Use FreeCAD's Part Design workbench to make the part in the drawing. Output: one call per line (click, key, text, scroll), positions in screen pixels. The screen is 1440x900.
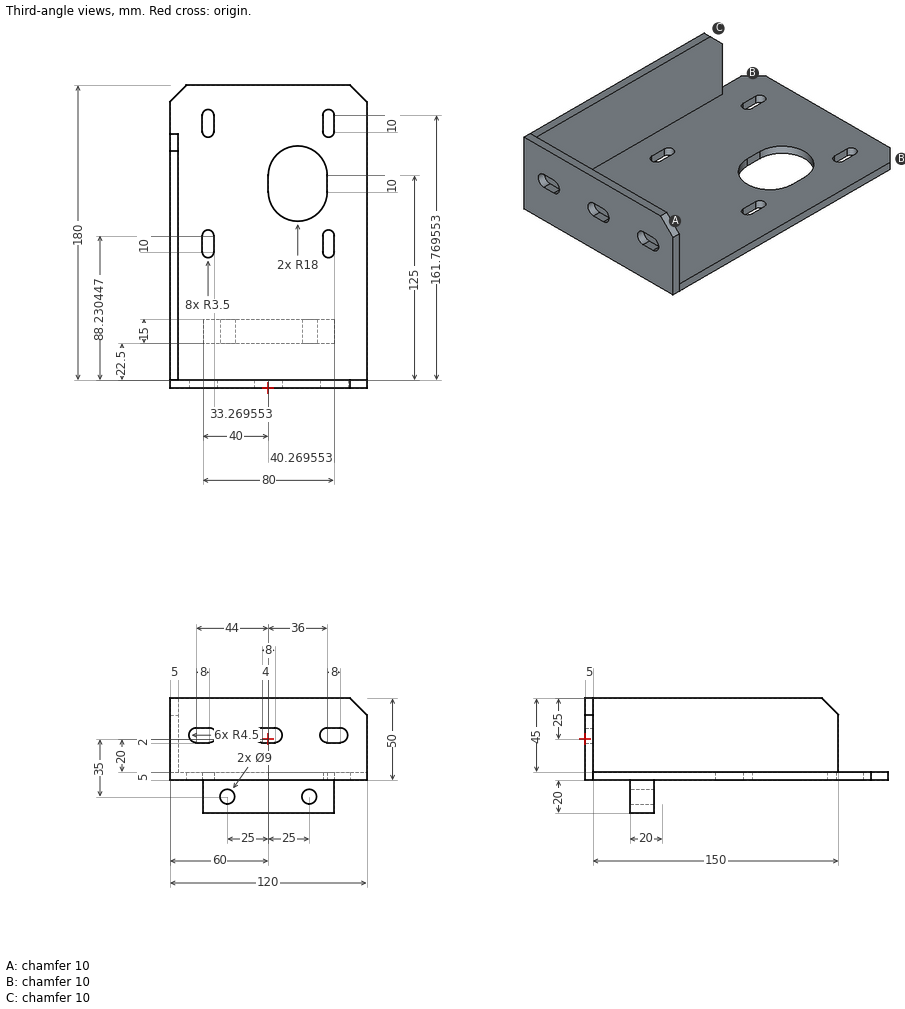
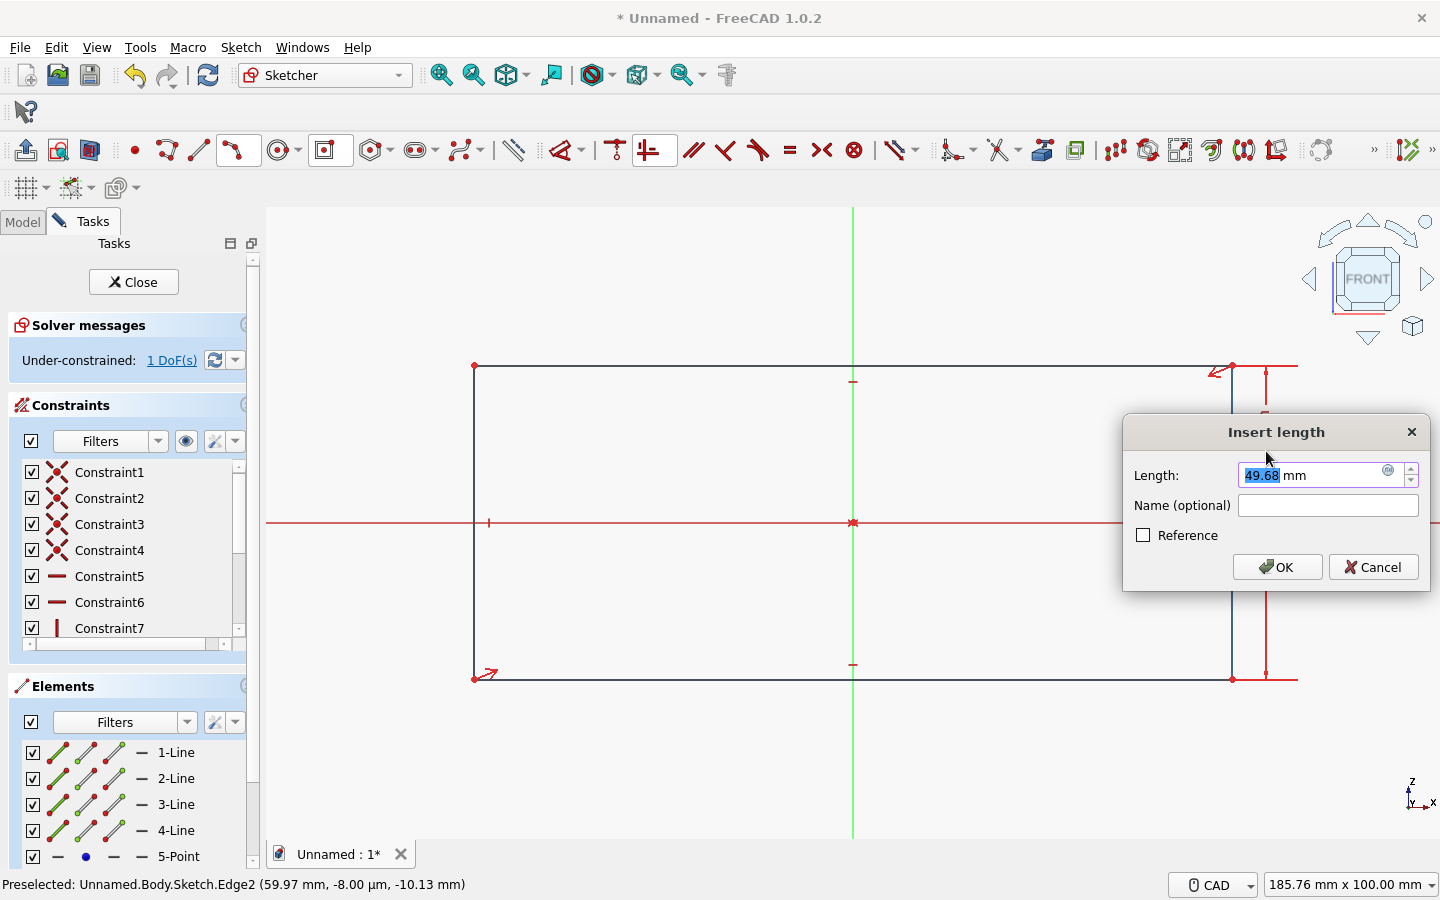
text(50)
key(Return)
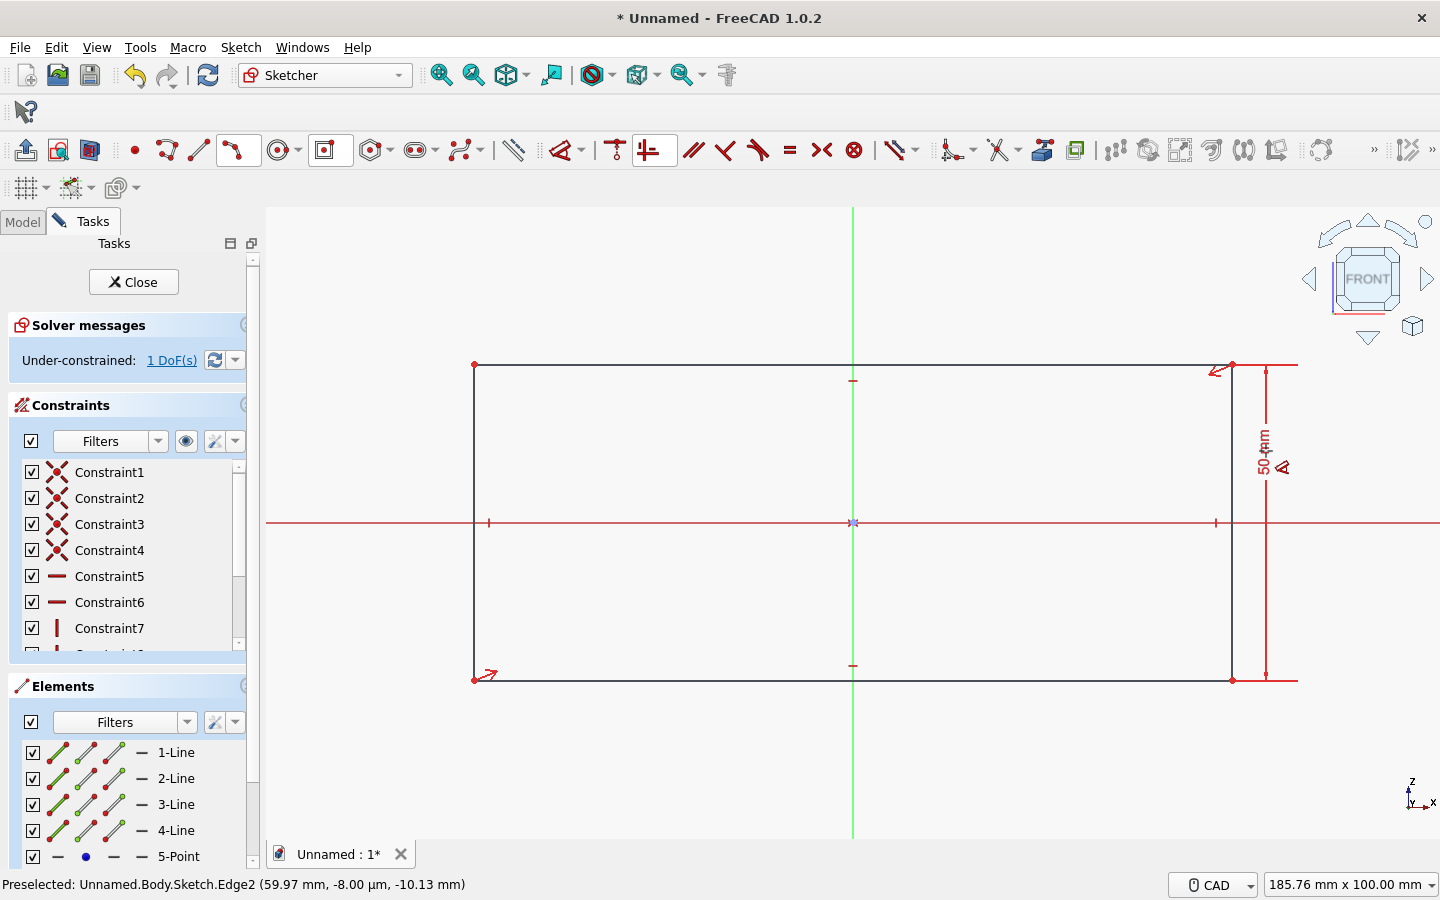
click(701, 681)
click(679, 715)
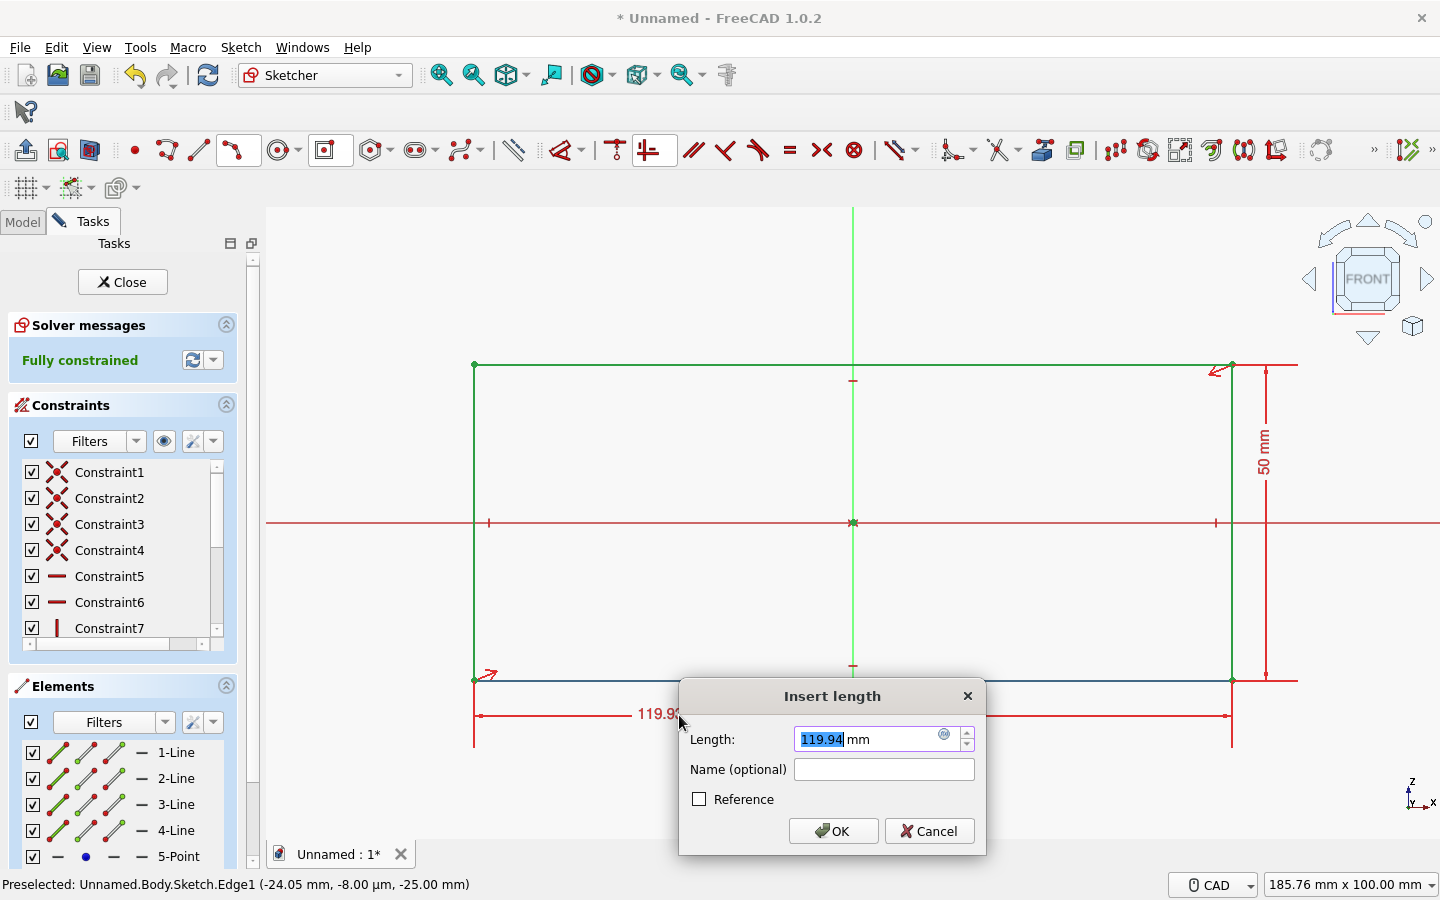
text(120)
key(Return)
key(Escape)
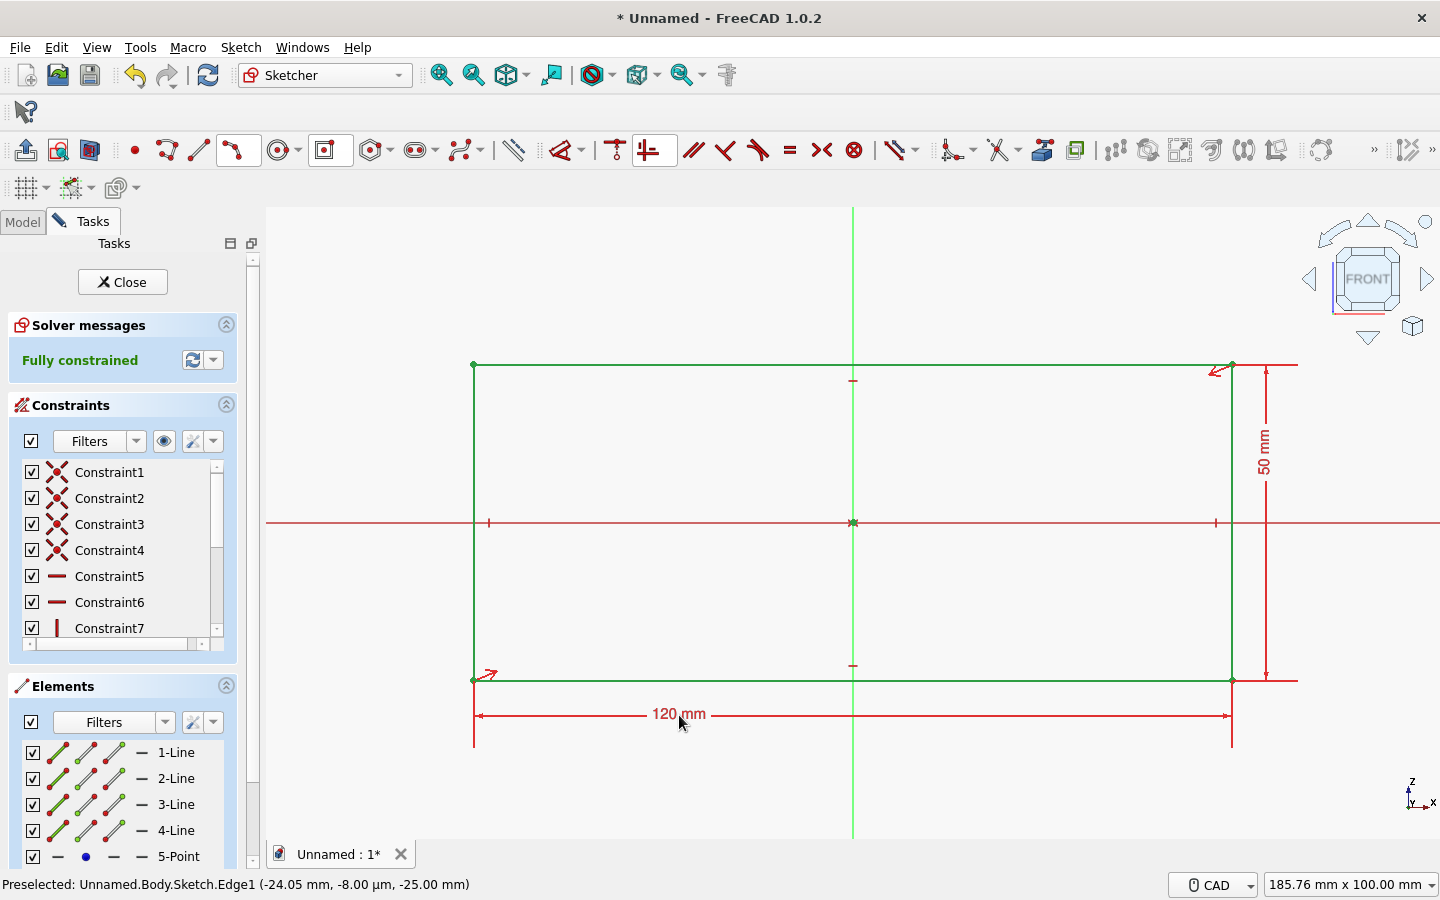
click(123, 282)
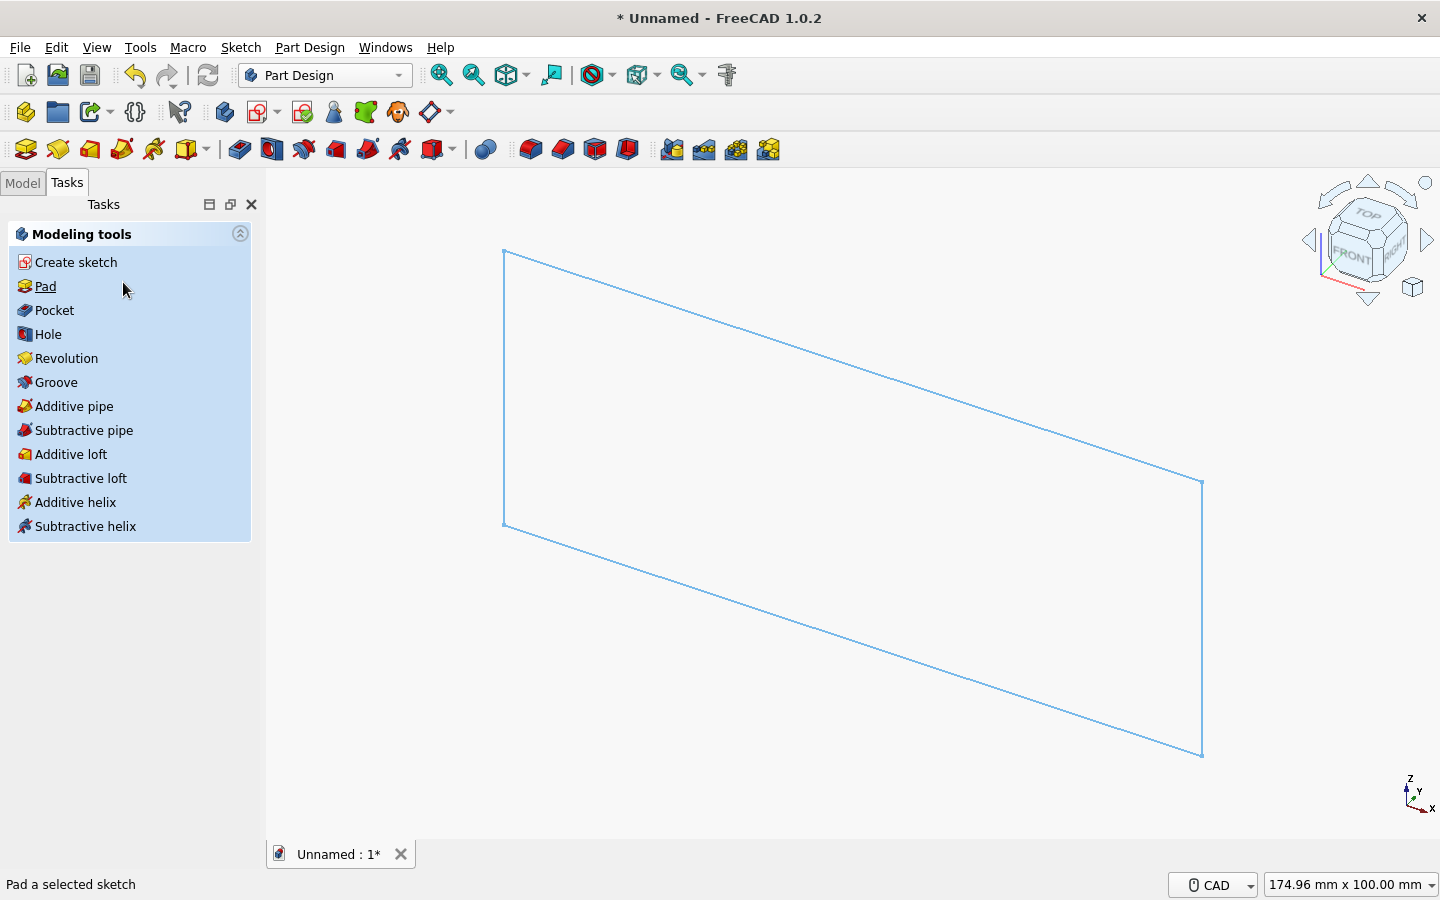
click(26, 150)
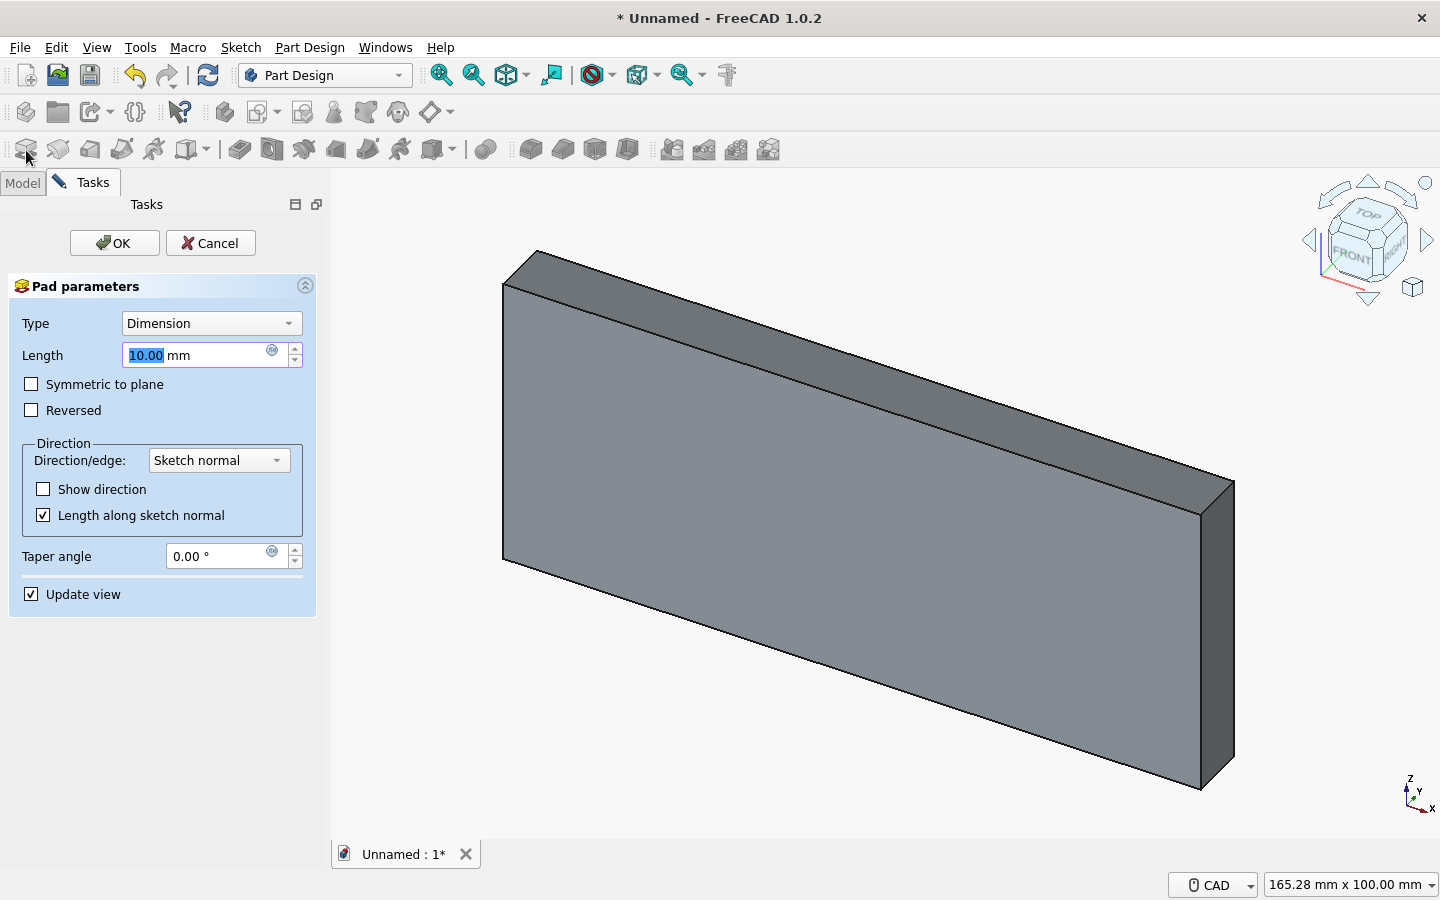
text(5)
key(Tab)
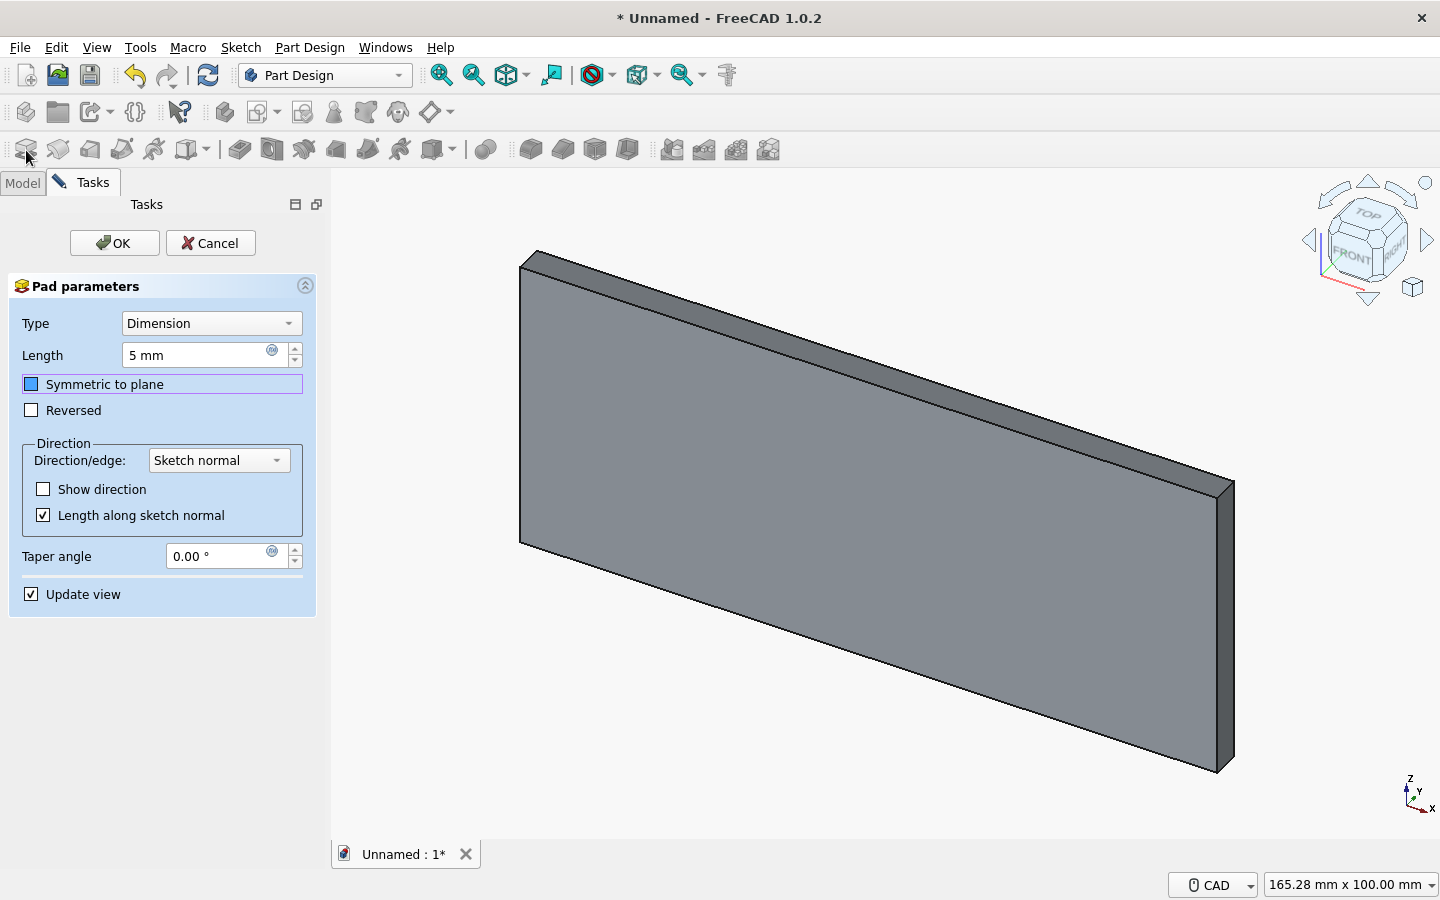
click(30, 410)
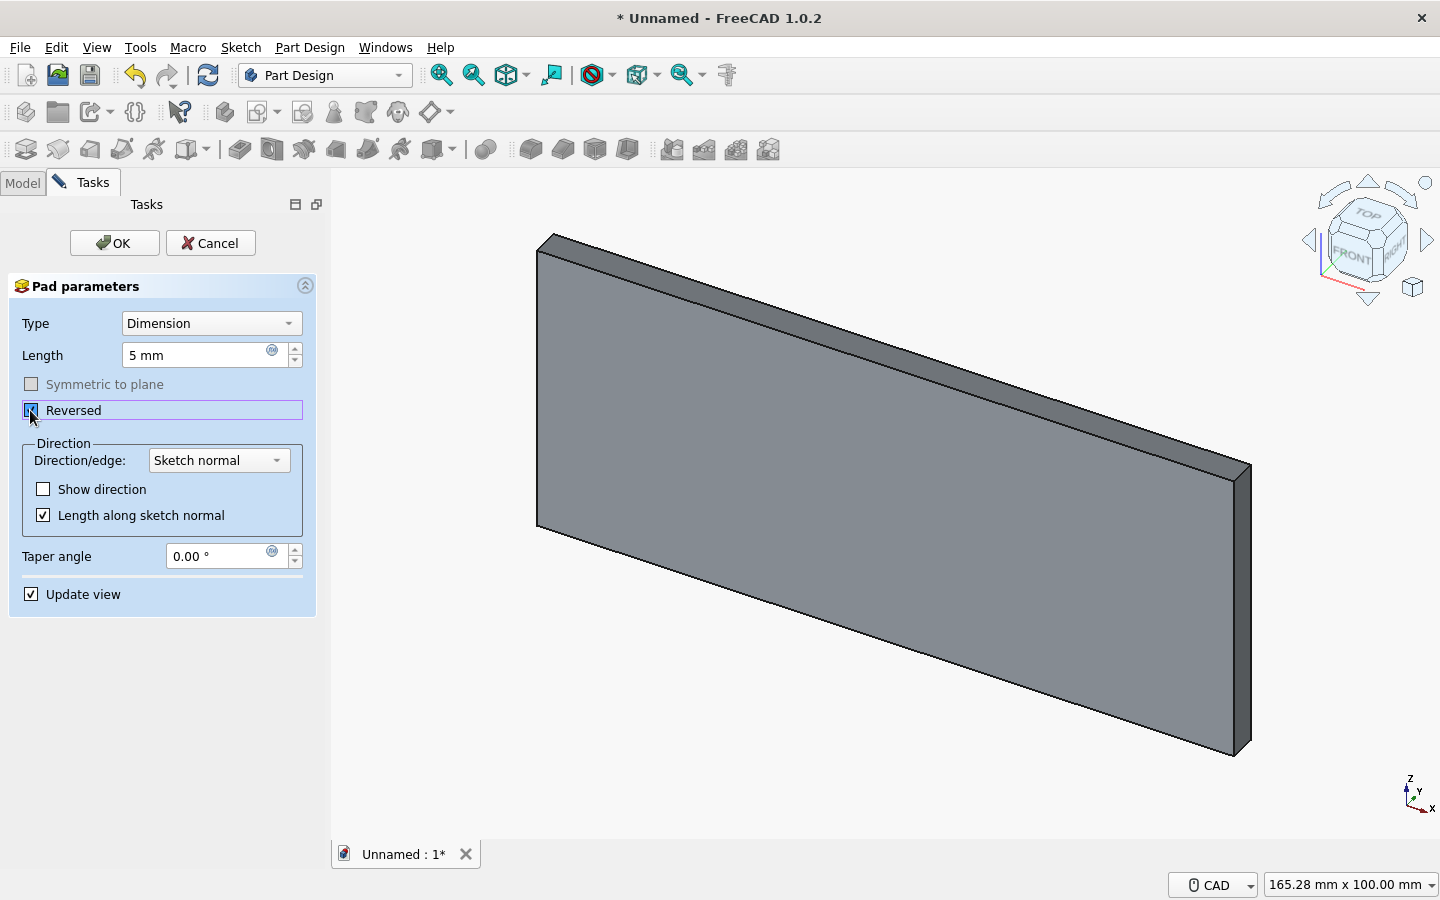
click(115, 243)